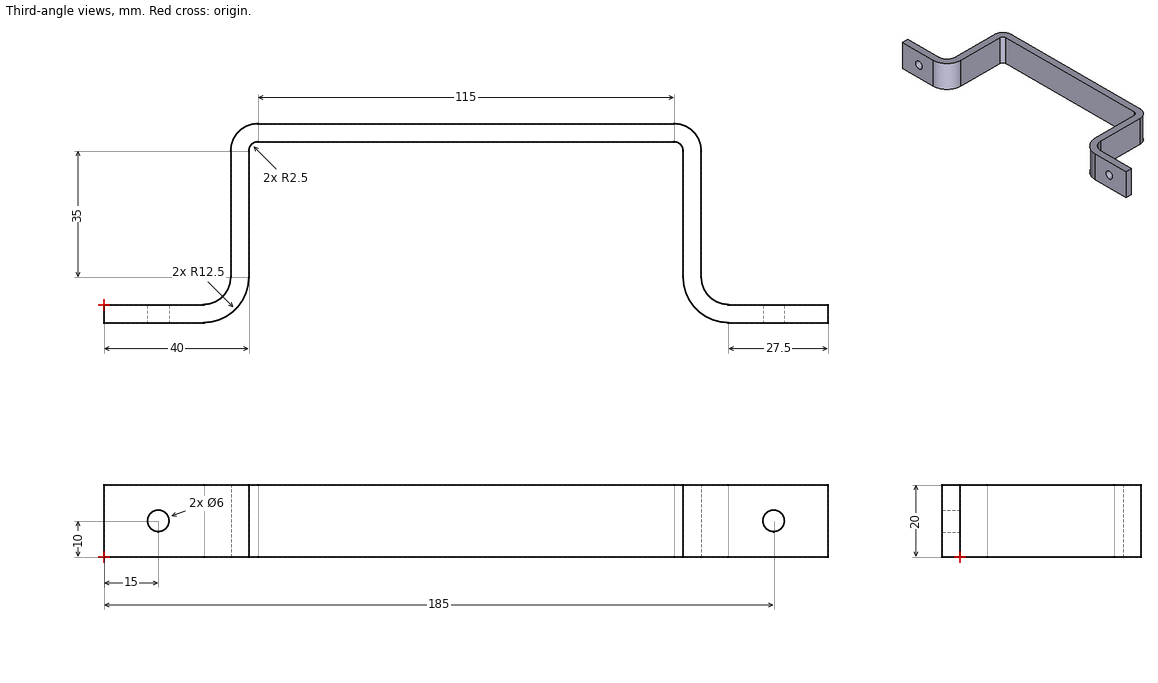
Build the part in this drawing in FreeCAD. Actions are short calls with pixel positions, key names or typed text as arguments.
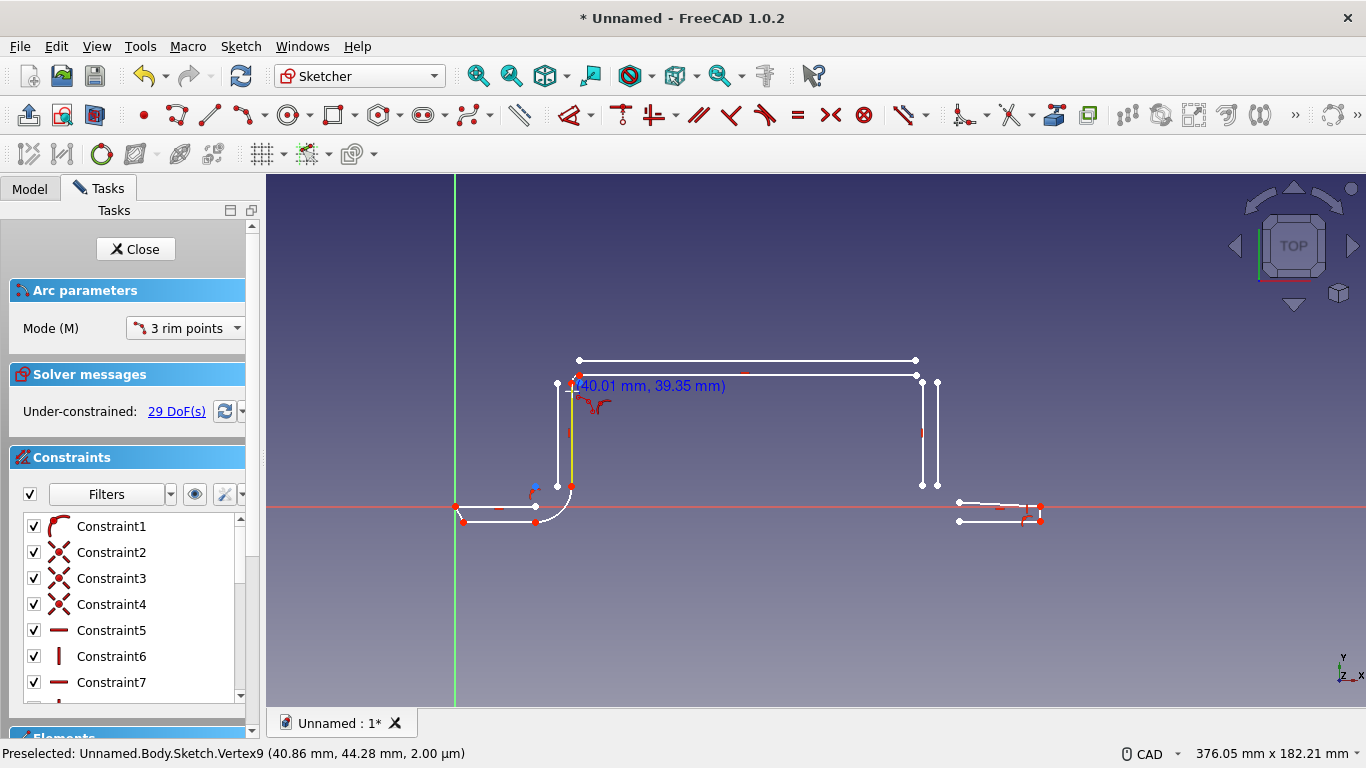
scroll(916, 375, up, 3)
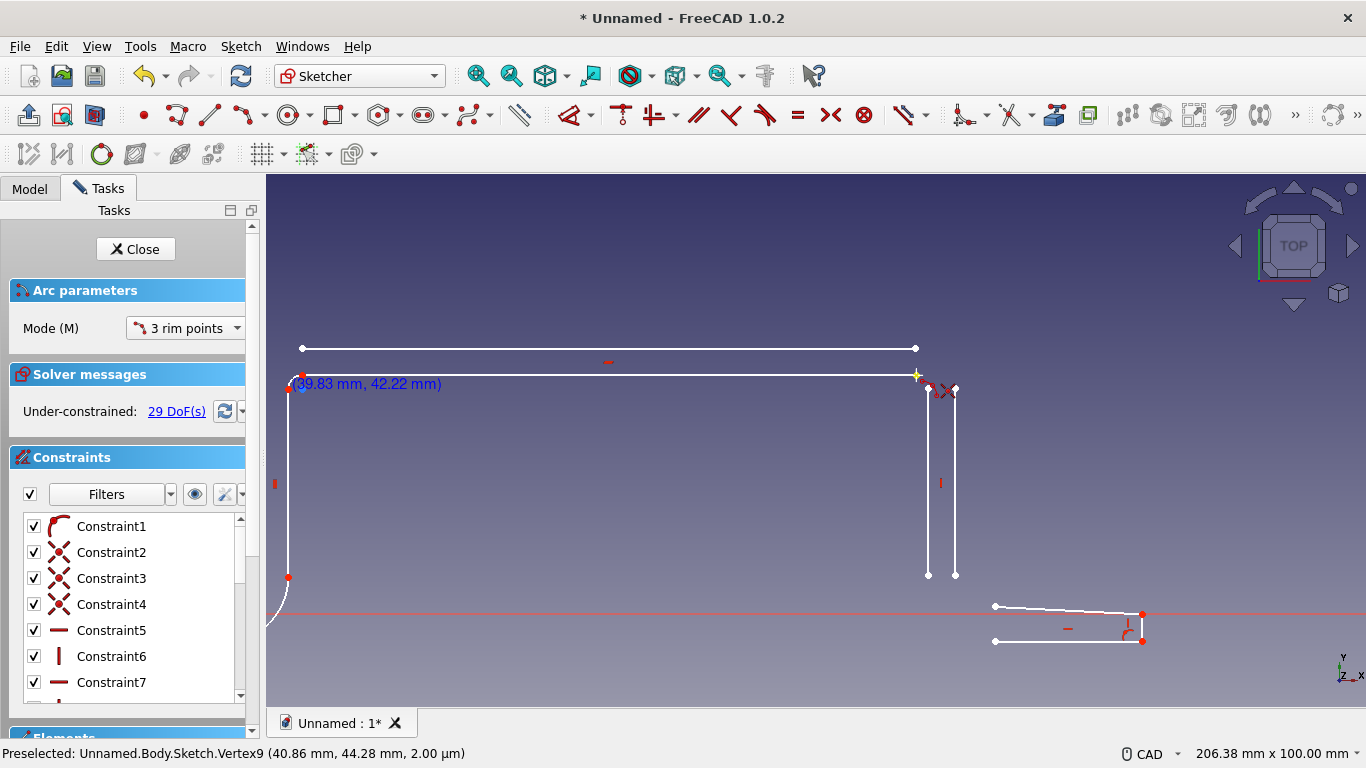
click(916, 375)
click(928, 389)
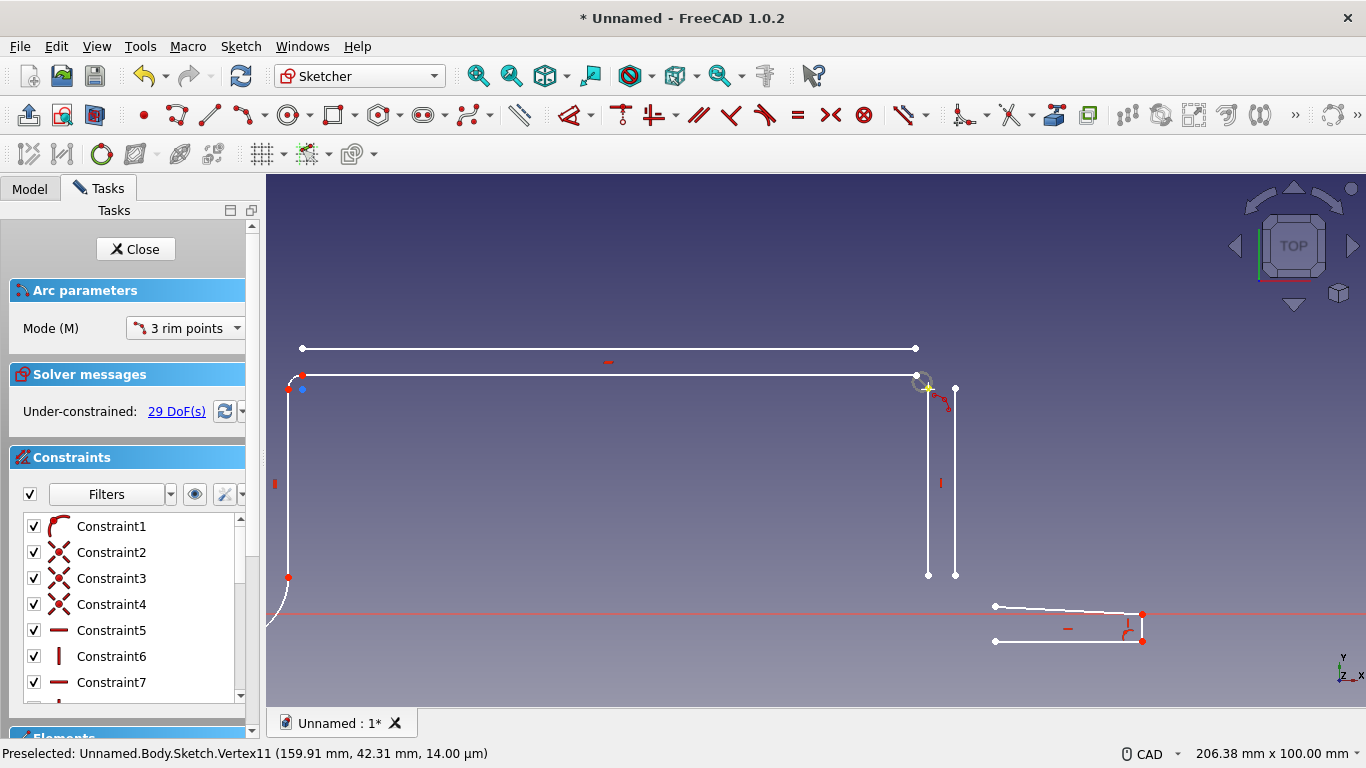
scroll(925, 379, up, 8)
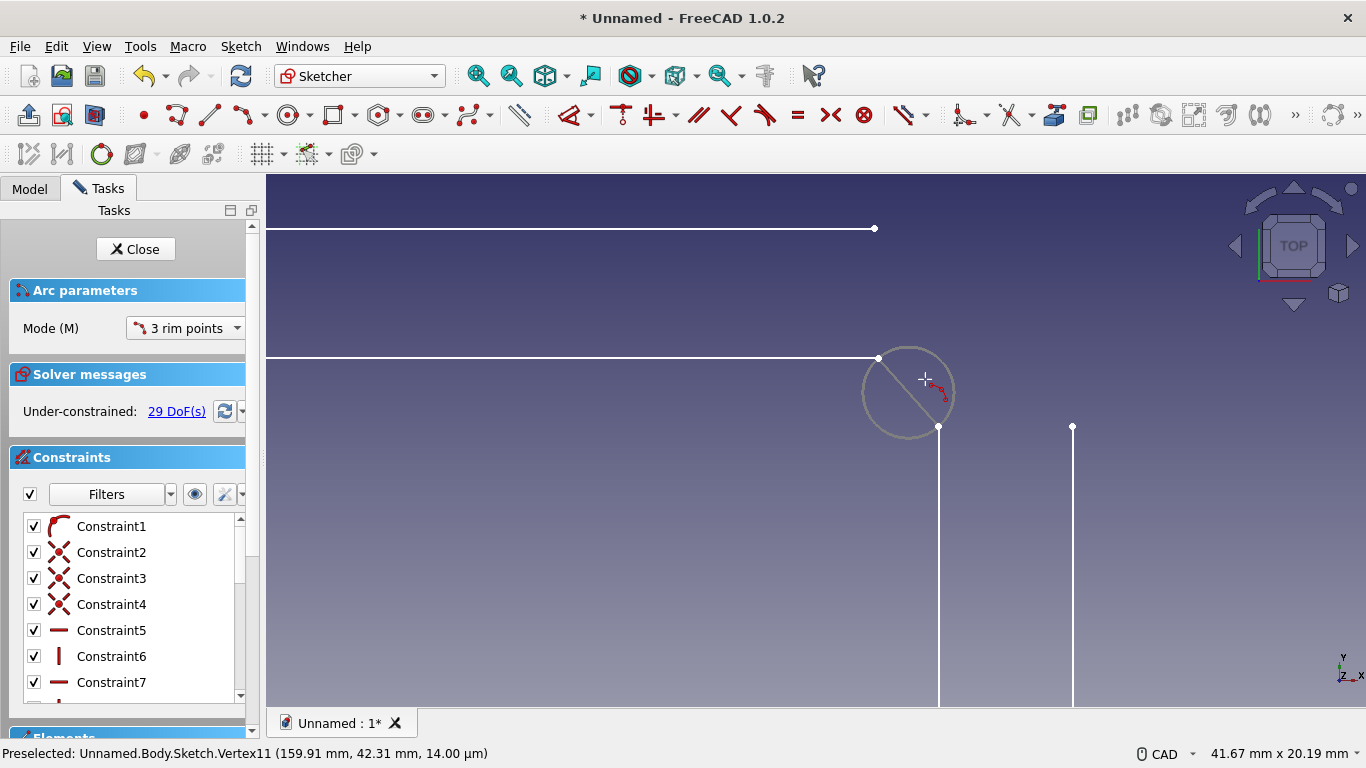
click(922, 375)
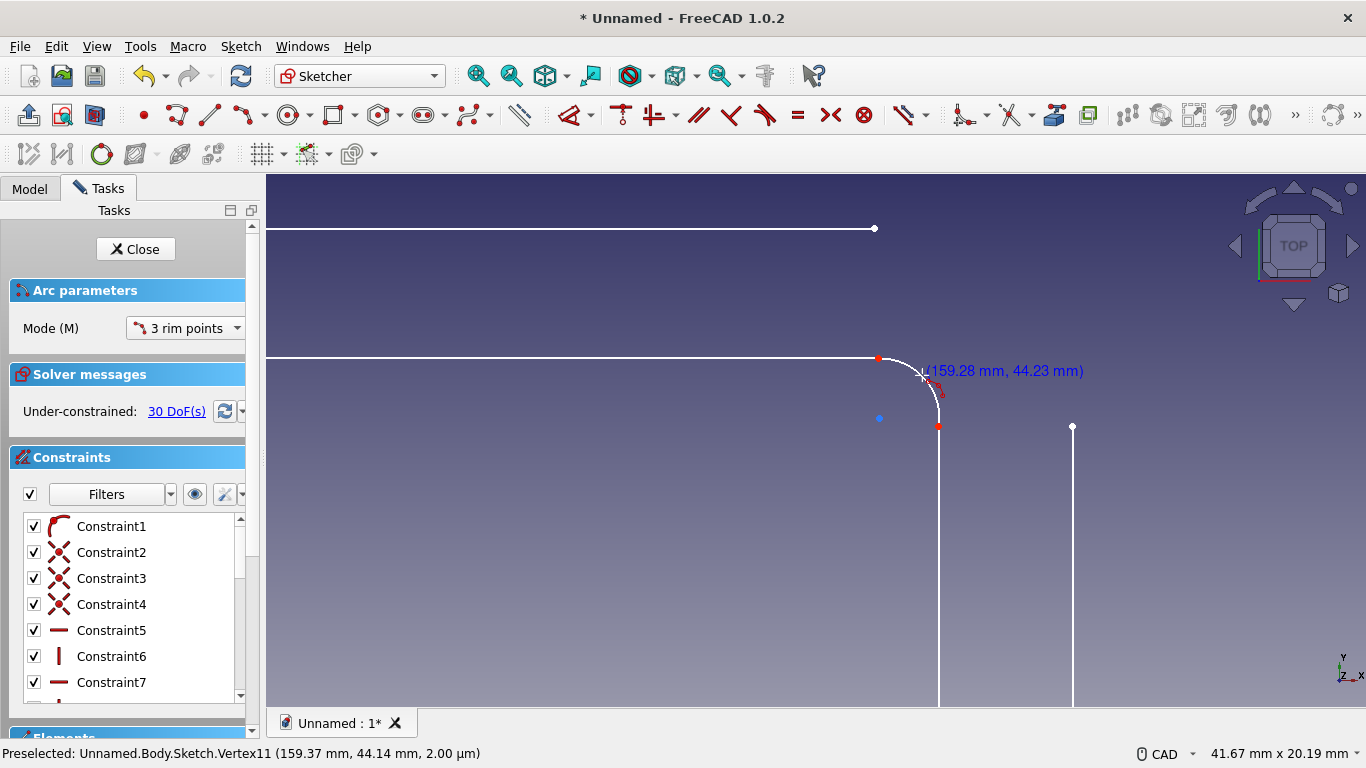
scroll(921, 377, down, 11)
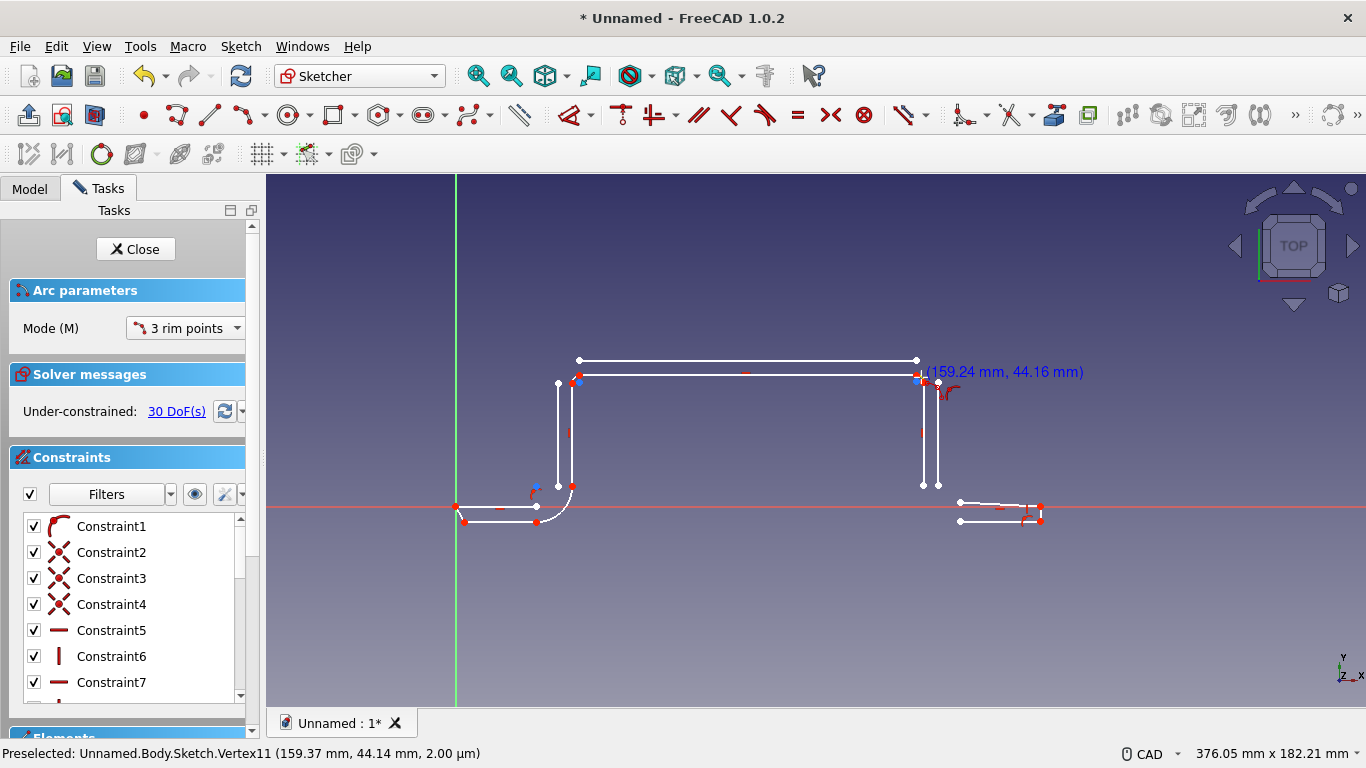
click(924, 485)
click(960, 522)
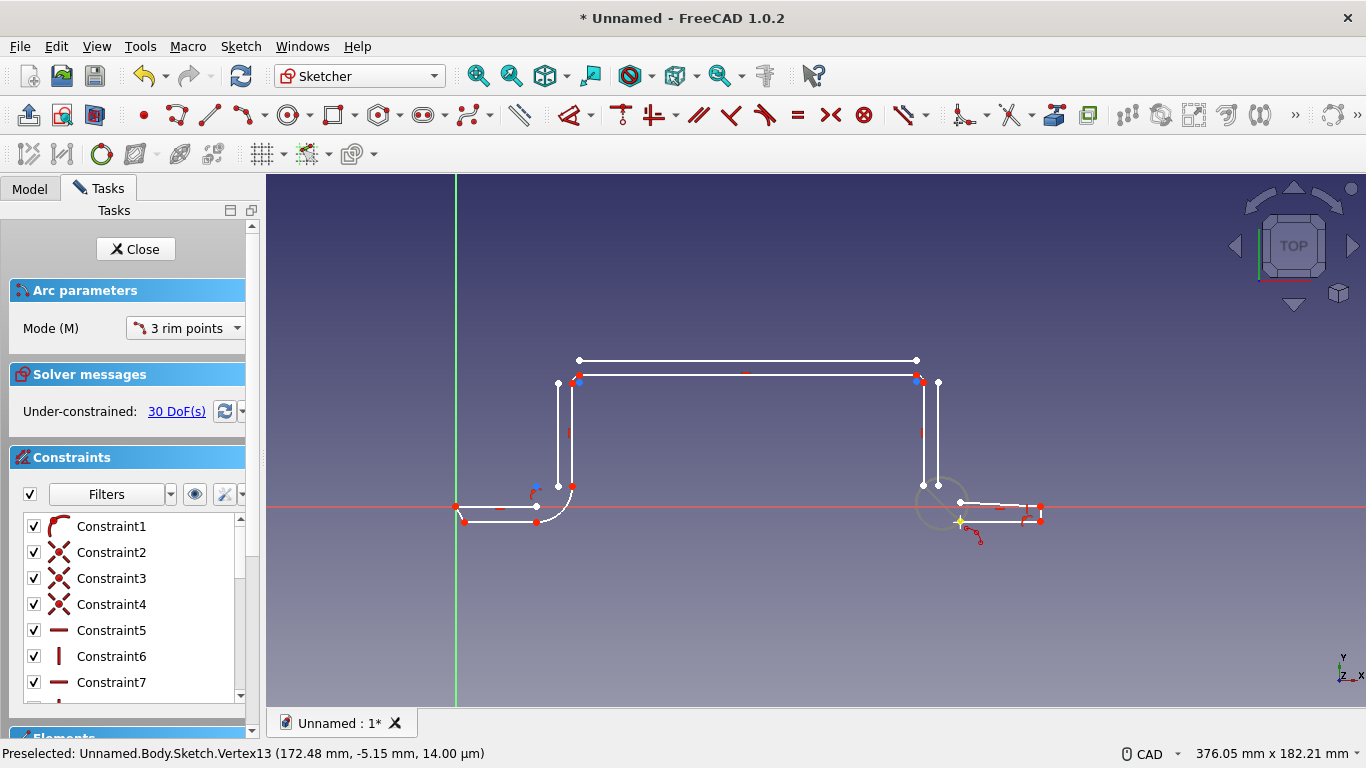
scroll(944, 517, up, 3)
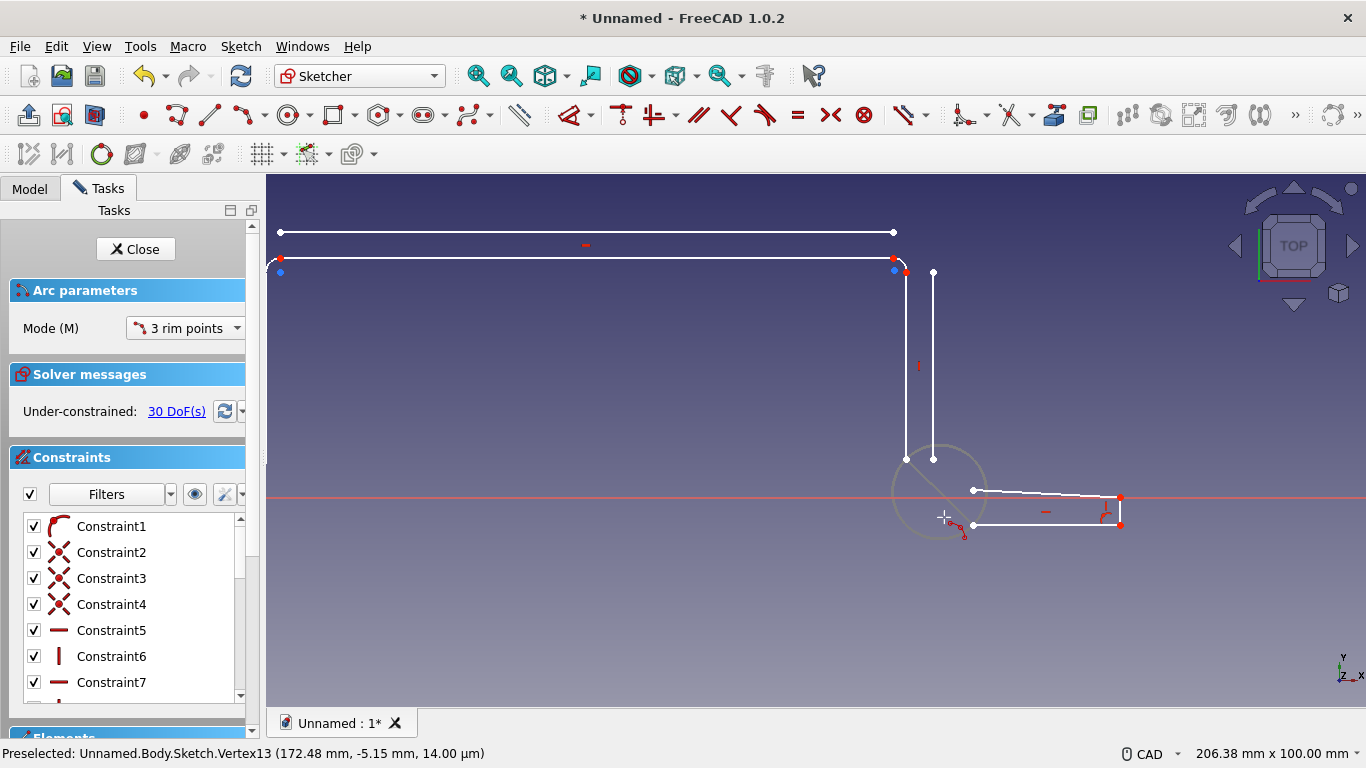
click(943, 517)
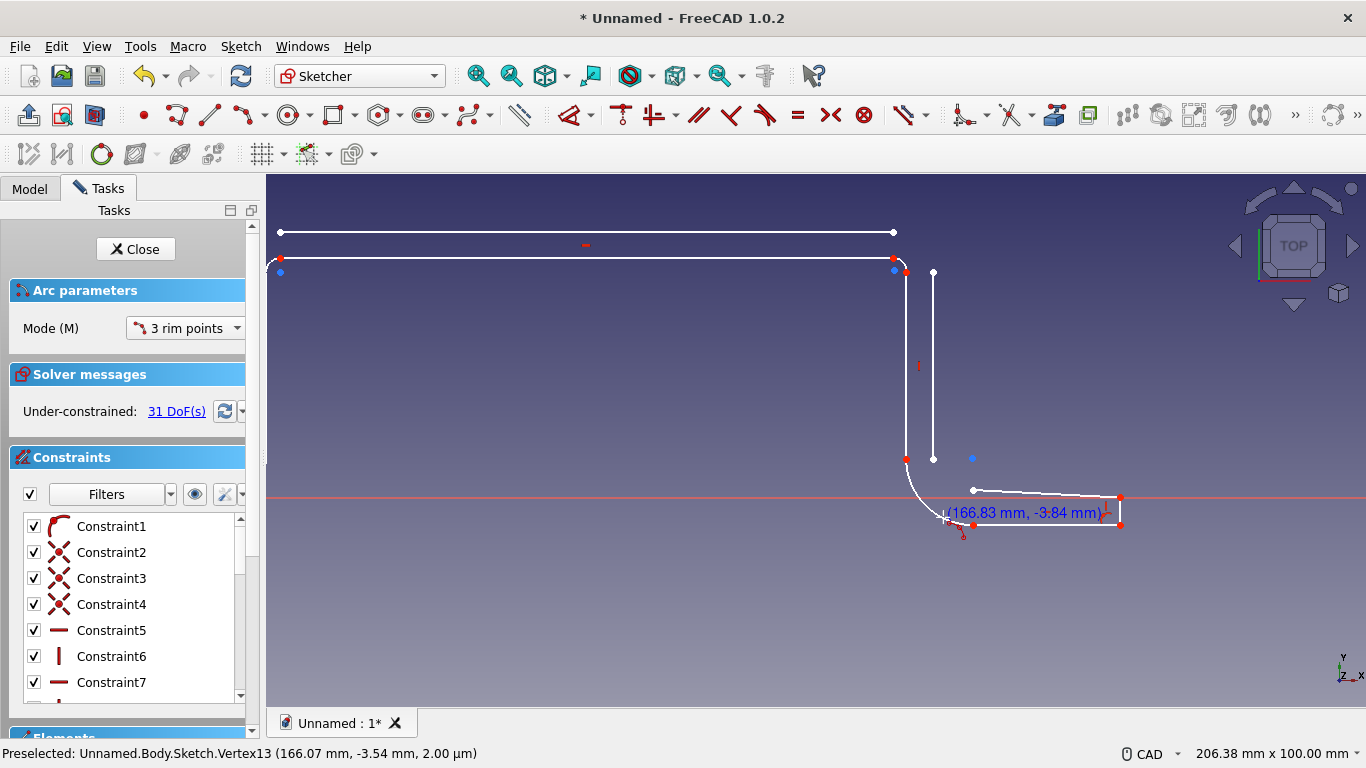
click(973, 490)
click(933, 459)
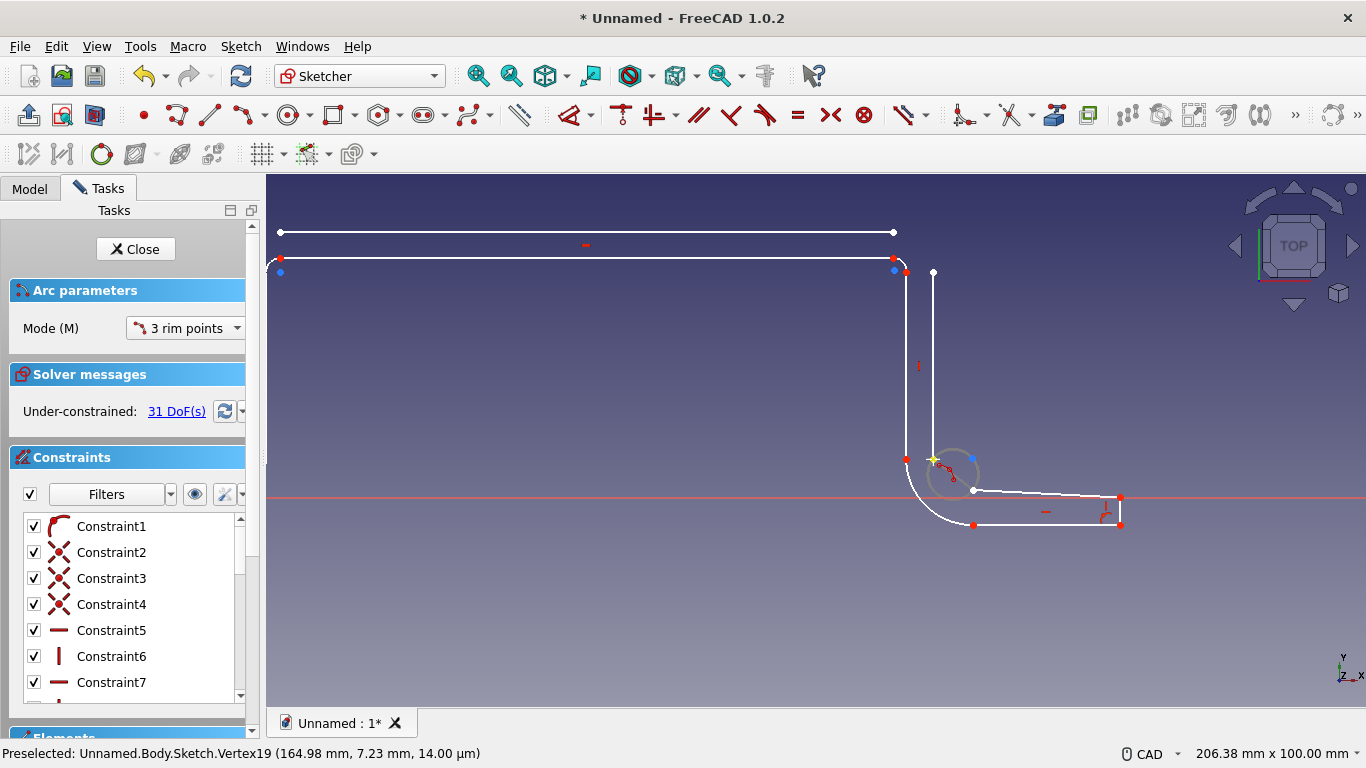
scroll(945, 486, up, 2)